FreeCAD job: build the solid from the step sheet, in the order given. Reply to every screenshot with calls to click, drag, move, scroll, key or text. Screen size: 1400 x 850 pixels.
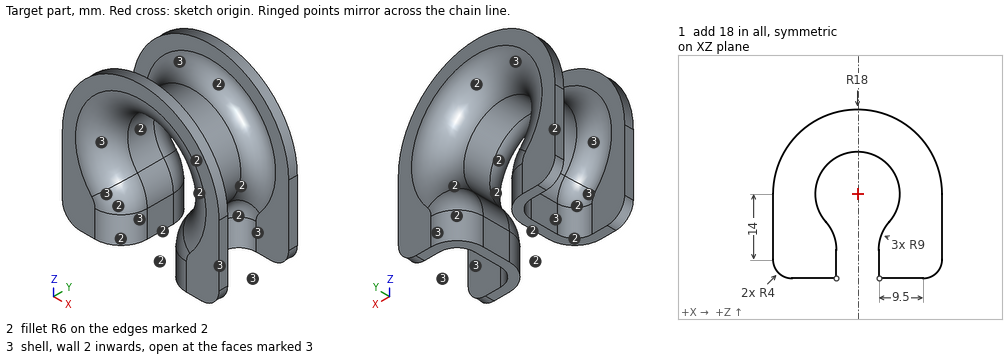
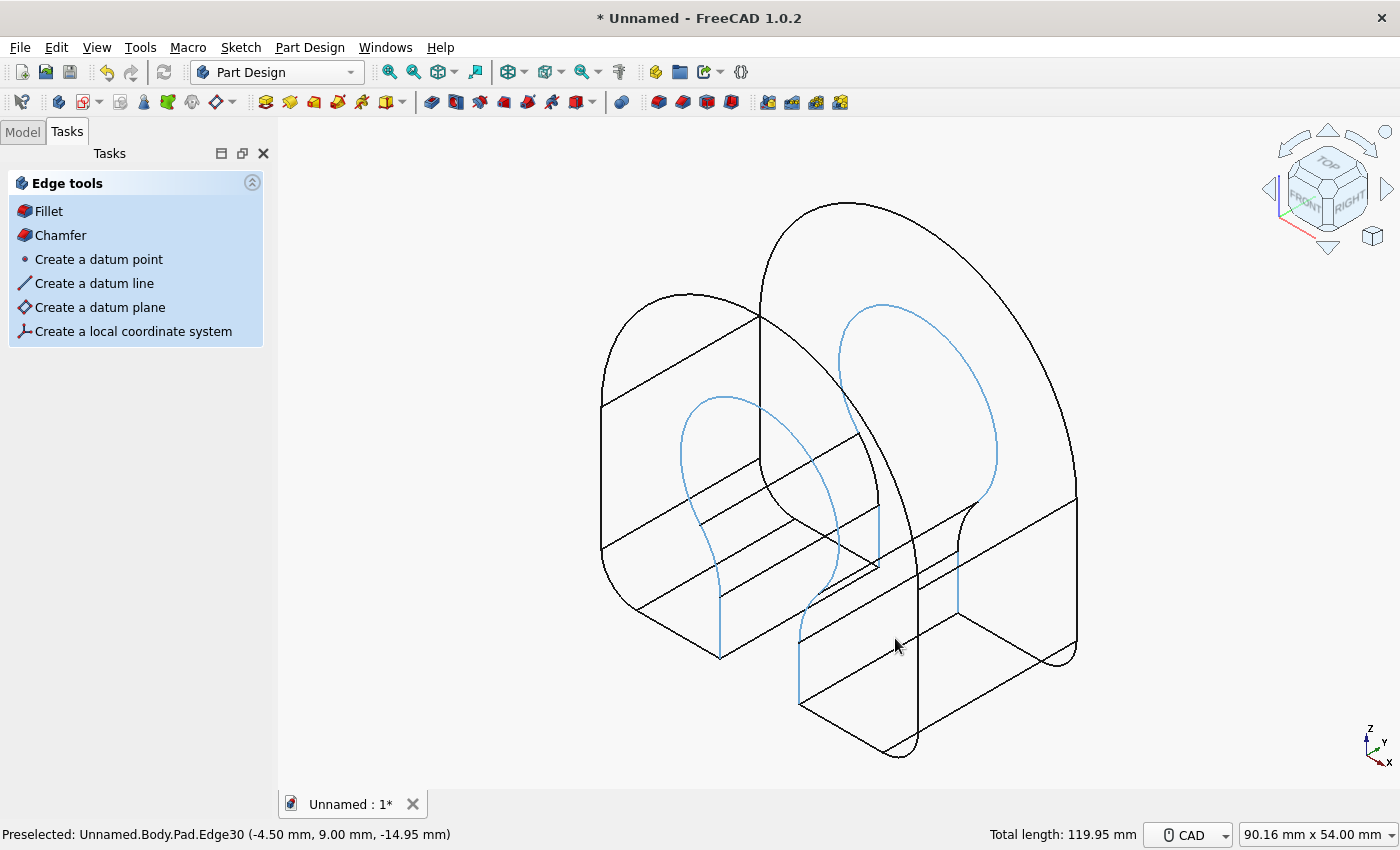
click(963, 521, ctrl)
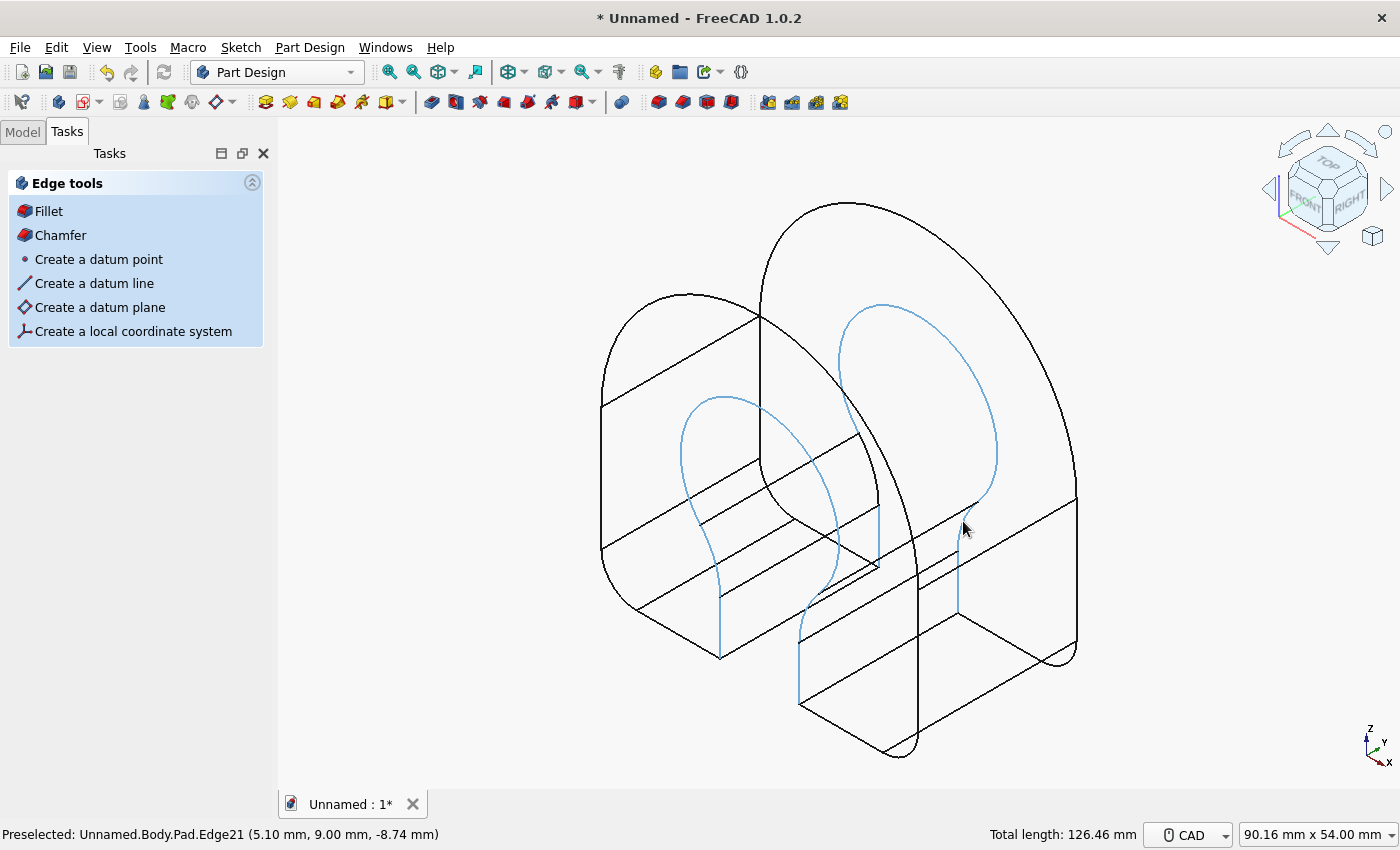
click(873, 469, ctrl)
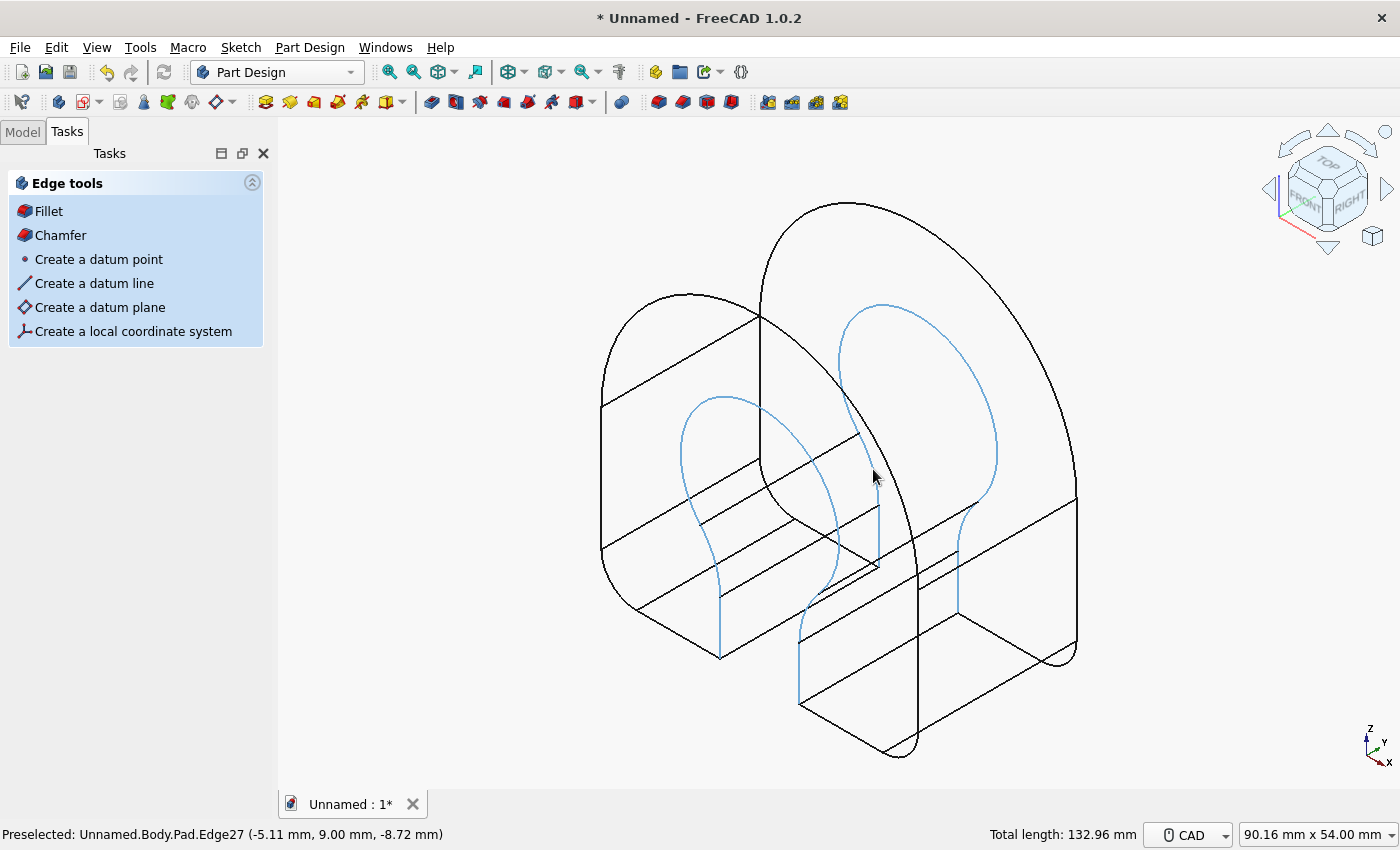
key(v)
key(1)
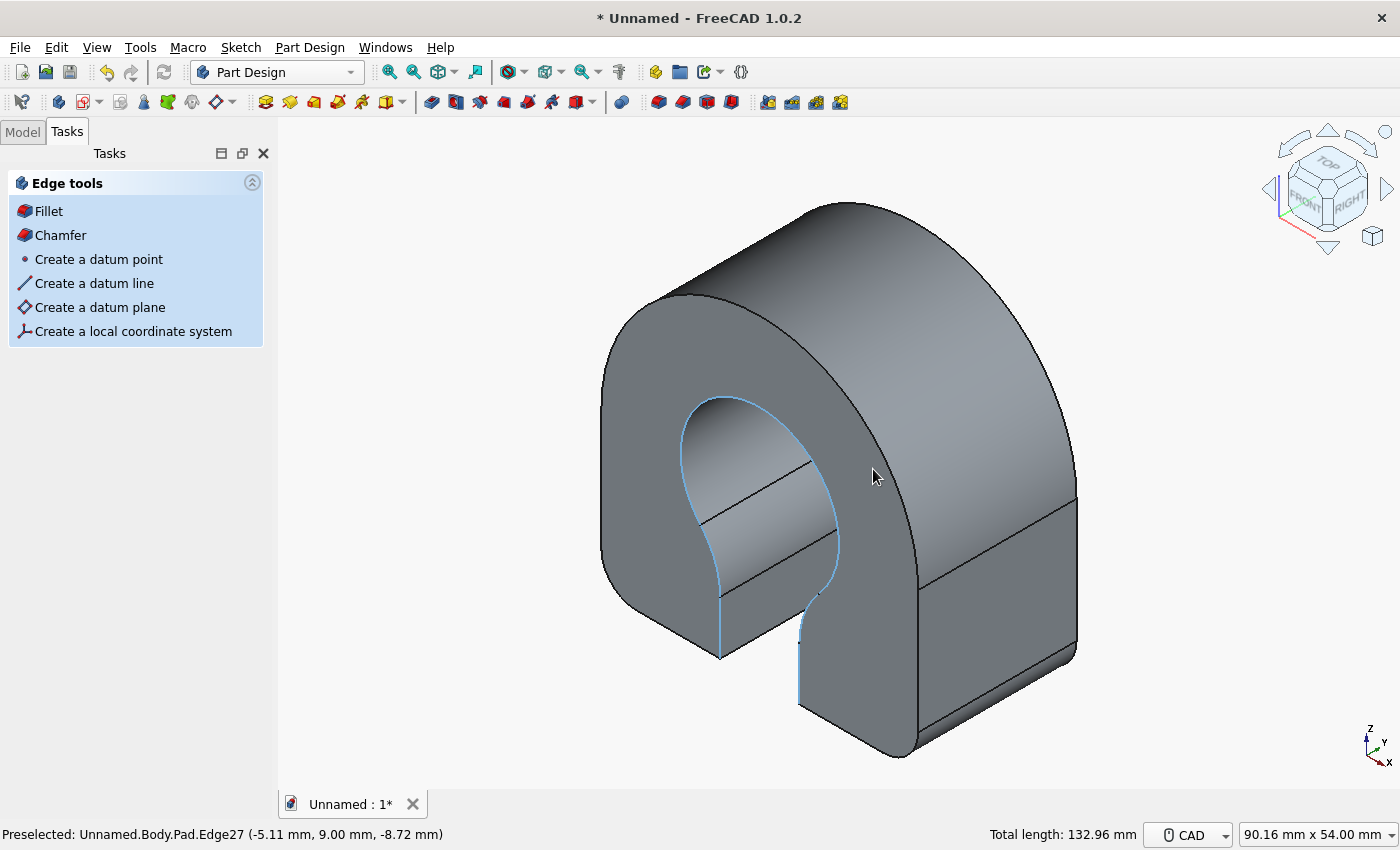
click(660, 102)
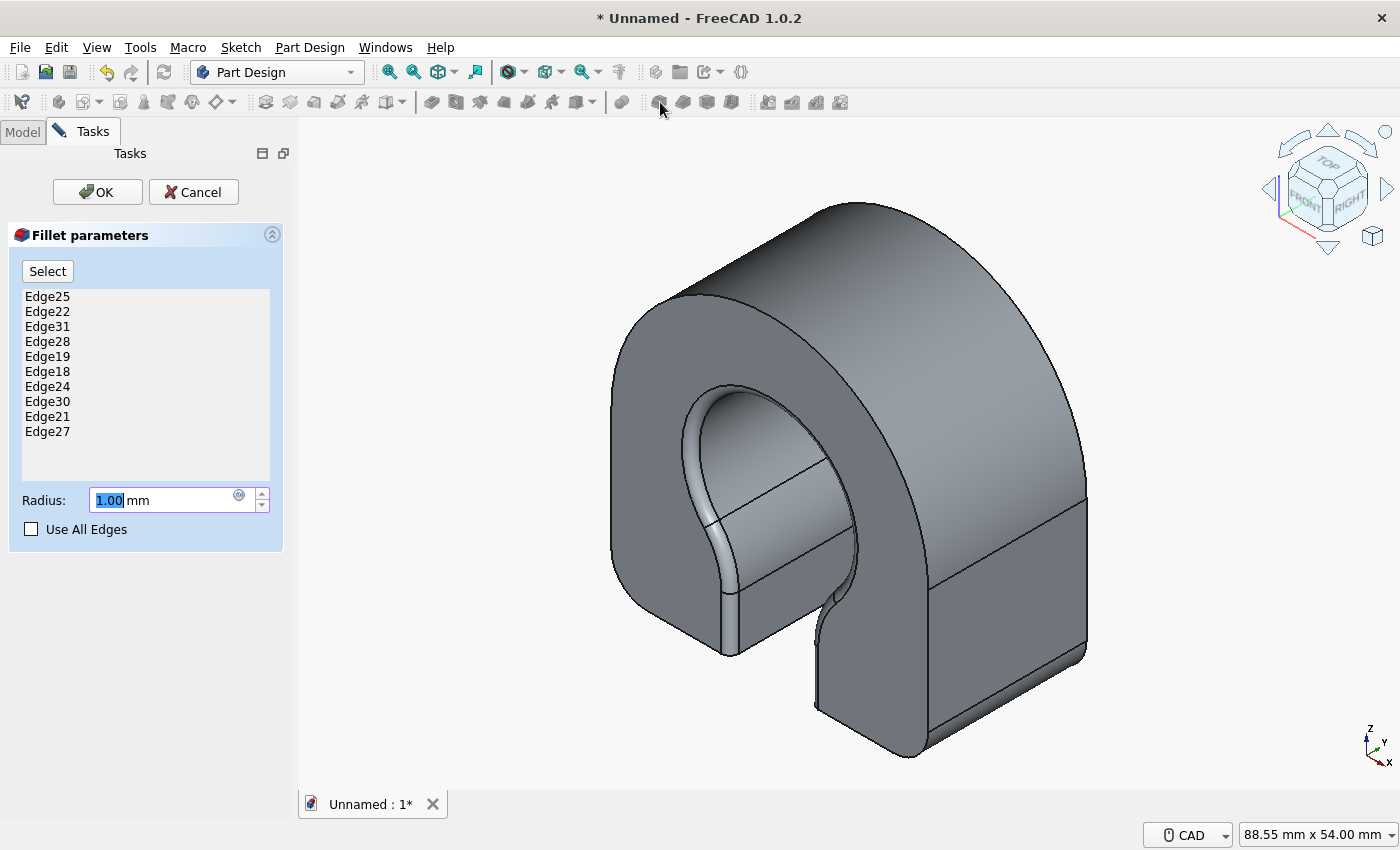
text(6)
key(Tab)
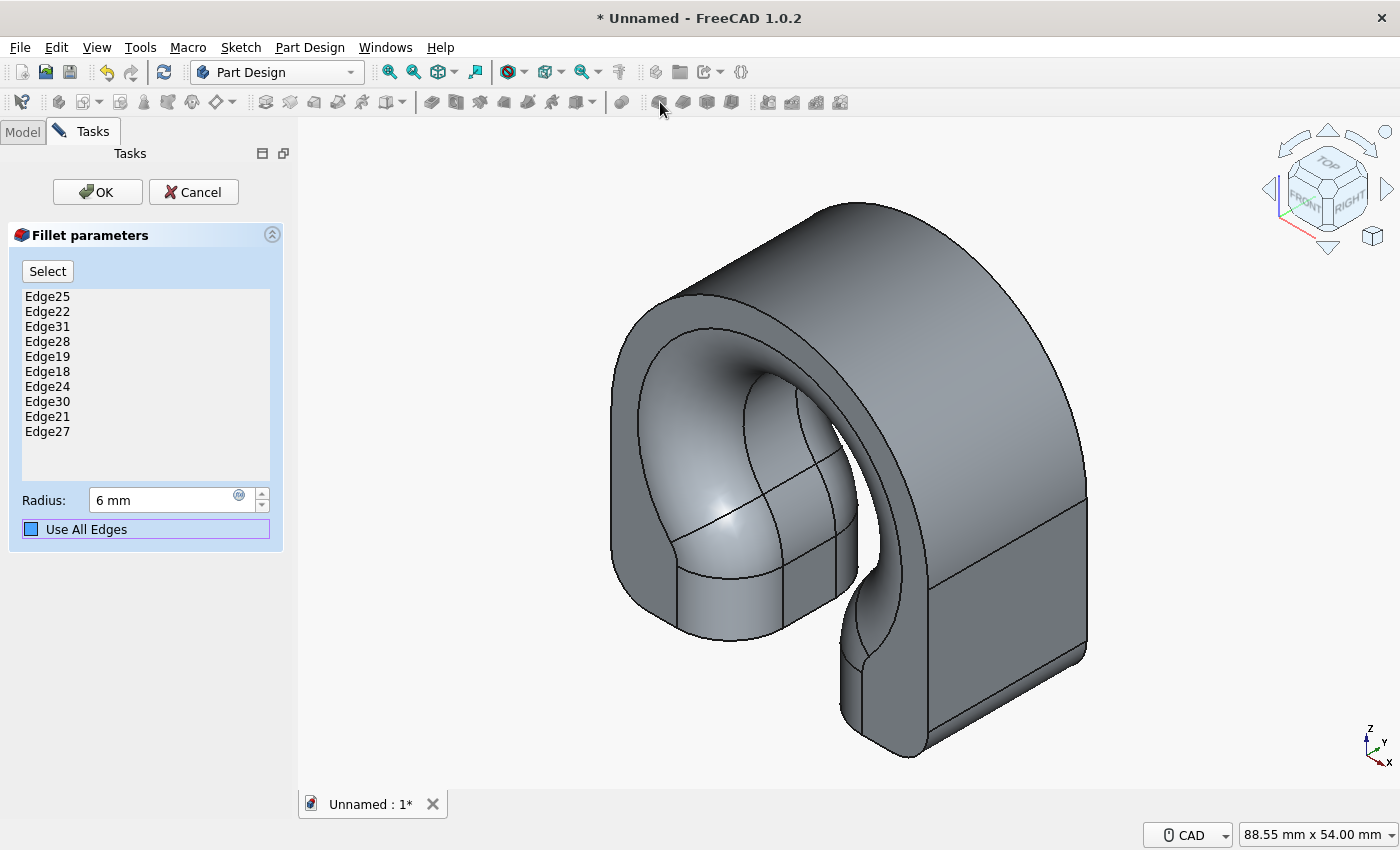
click(98, 192)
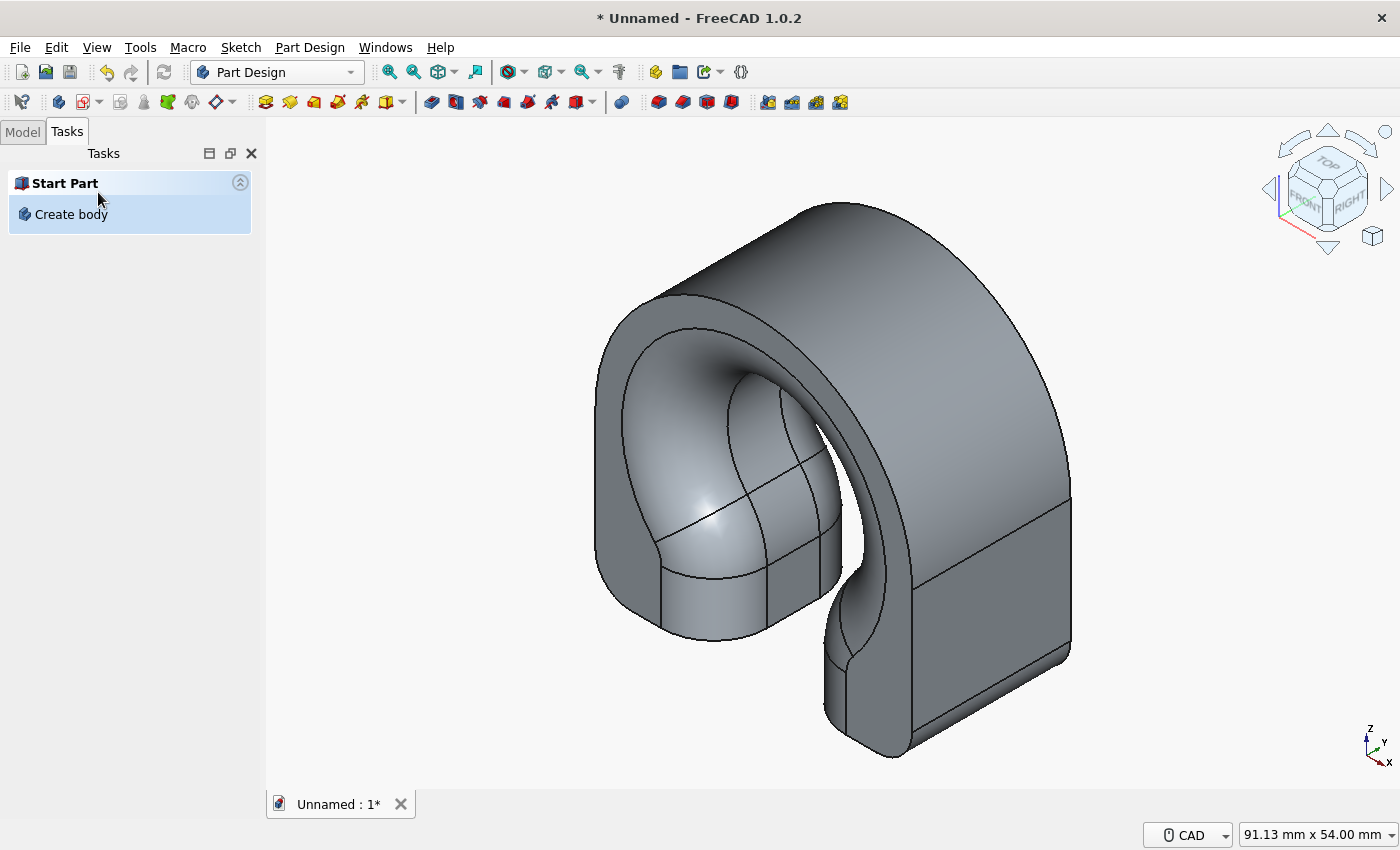
click(902, 327)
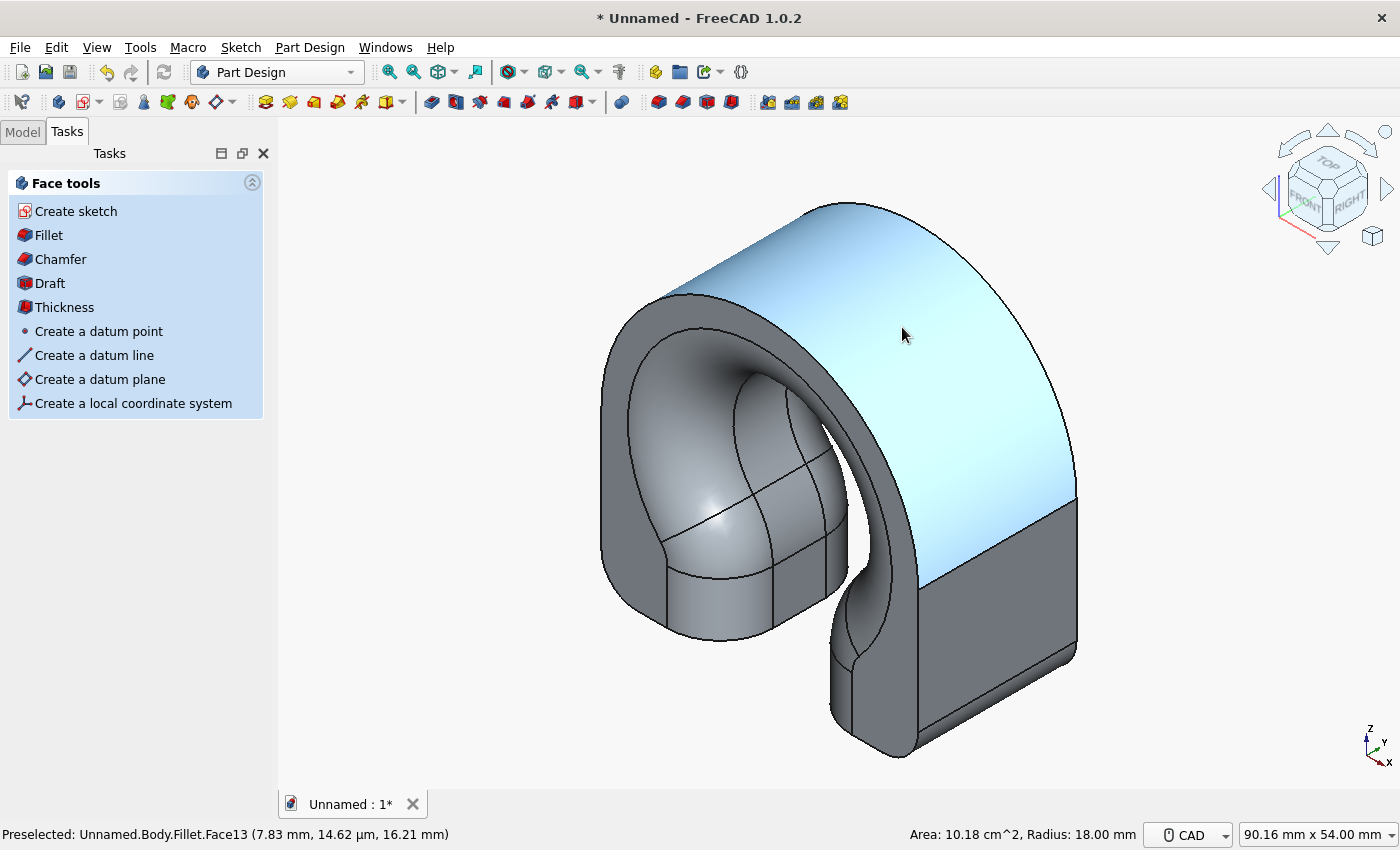
click(997, 615, ctrl)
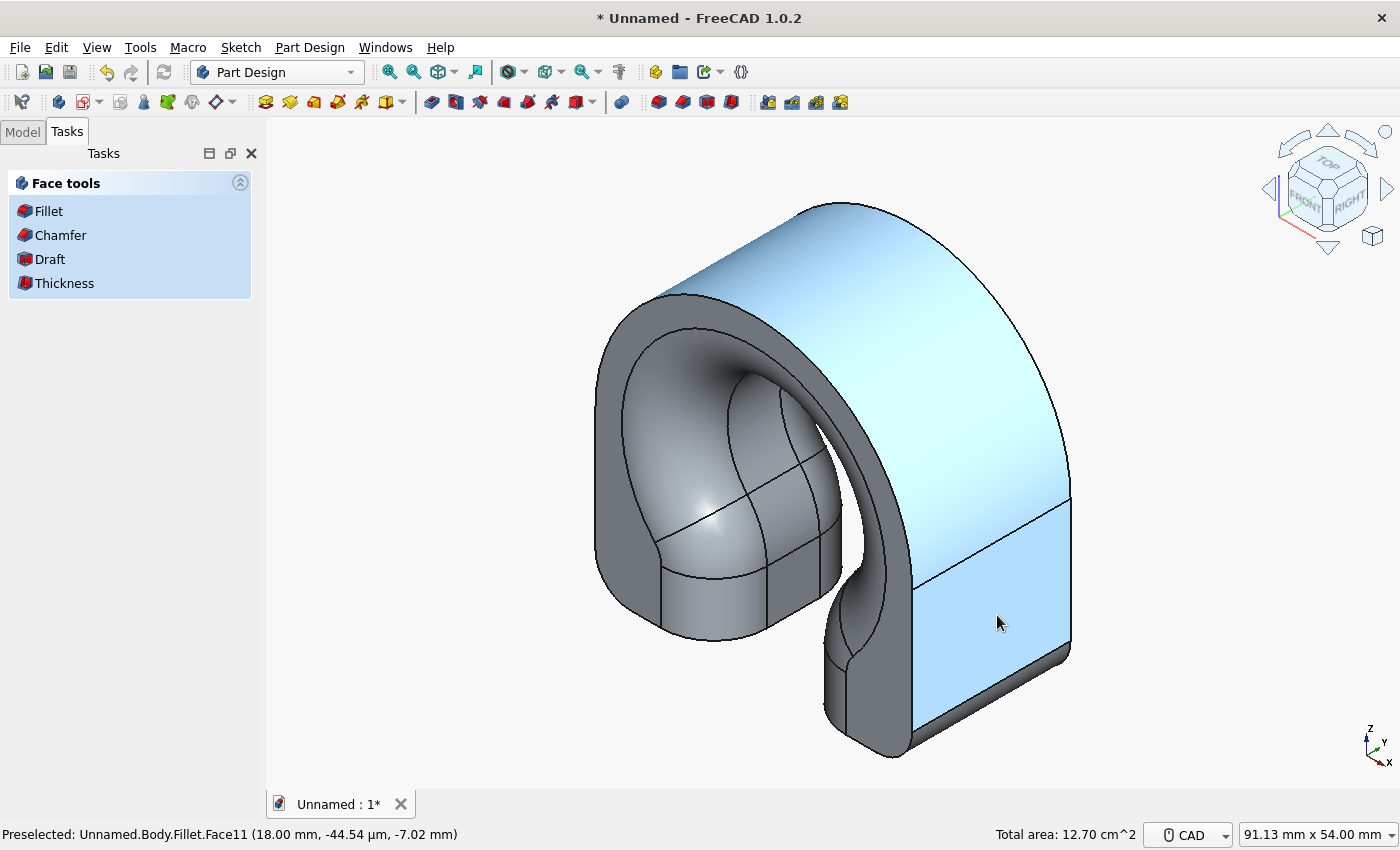
key(2)